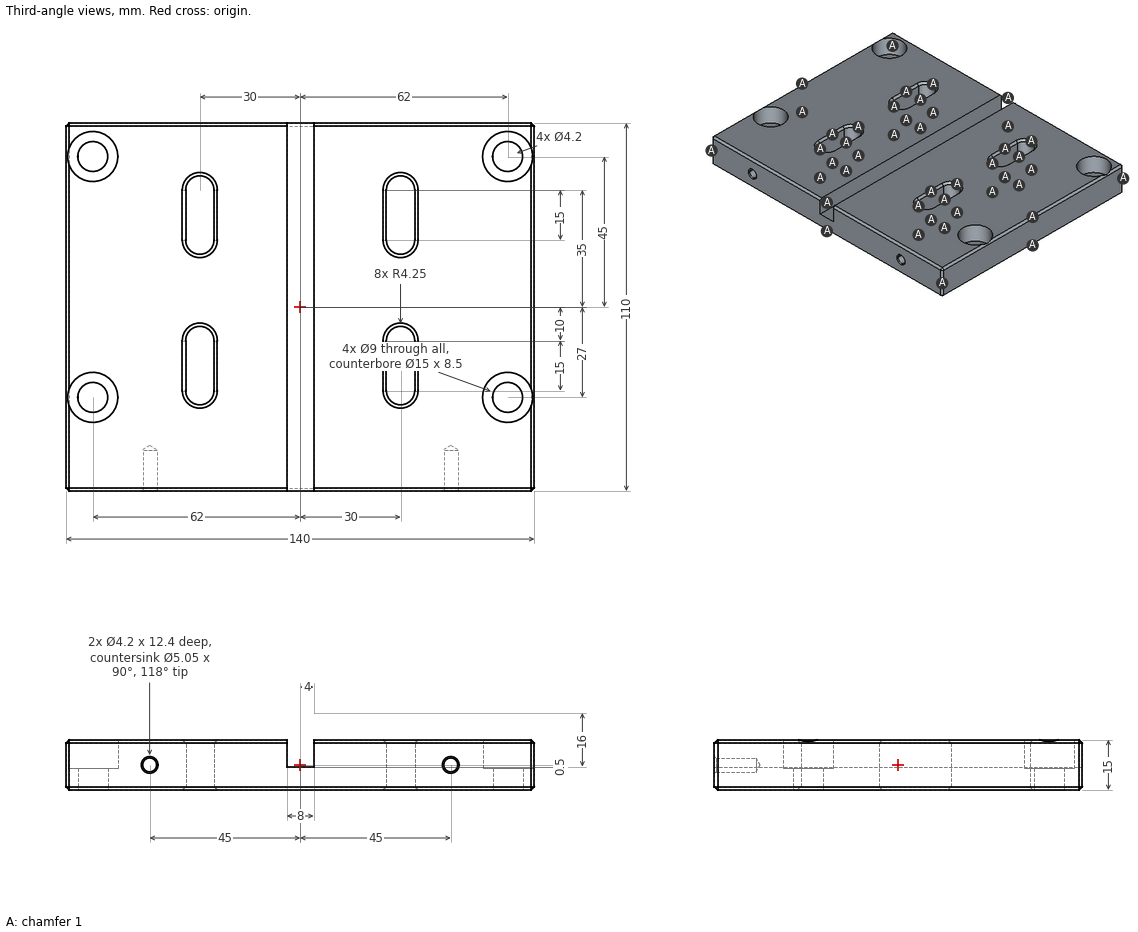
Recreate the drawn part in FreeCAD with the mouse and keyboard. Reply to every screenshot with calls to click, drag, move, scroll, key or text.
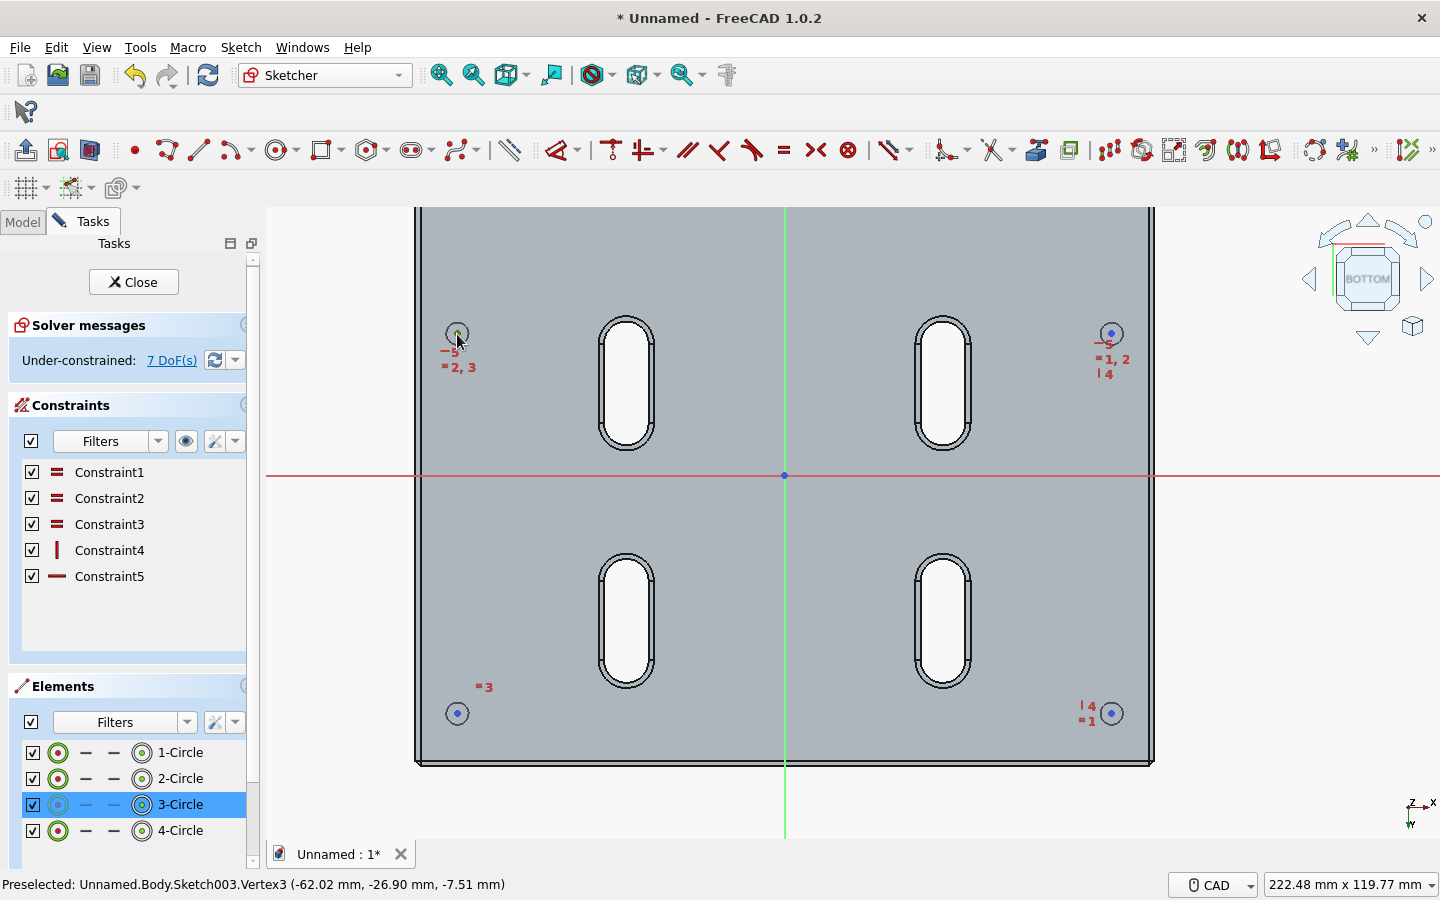
click(457, 714)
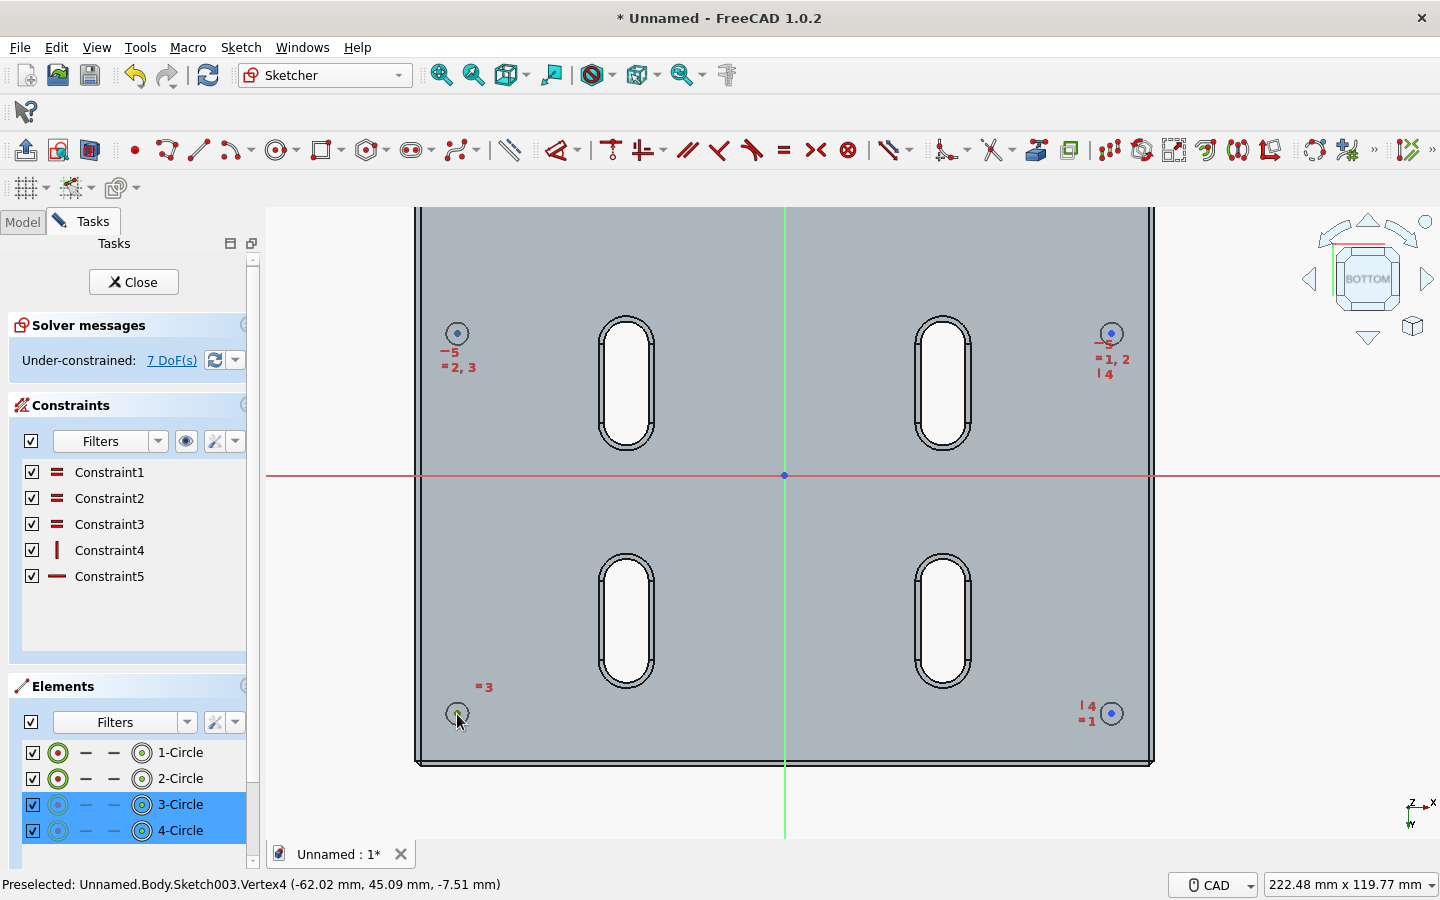
key(v)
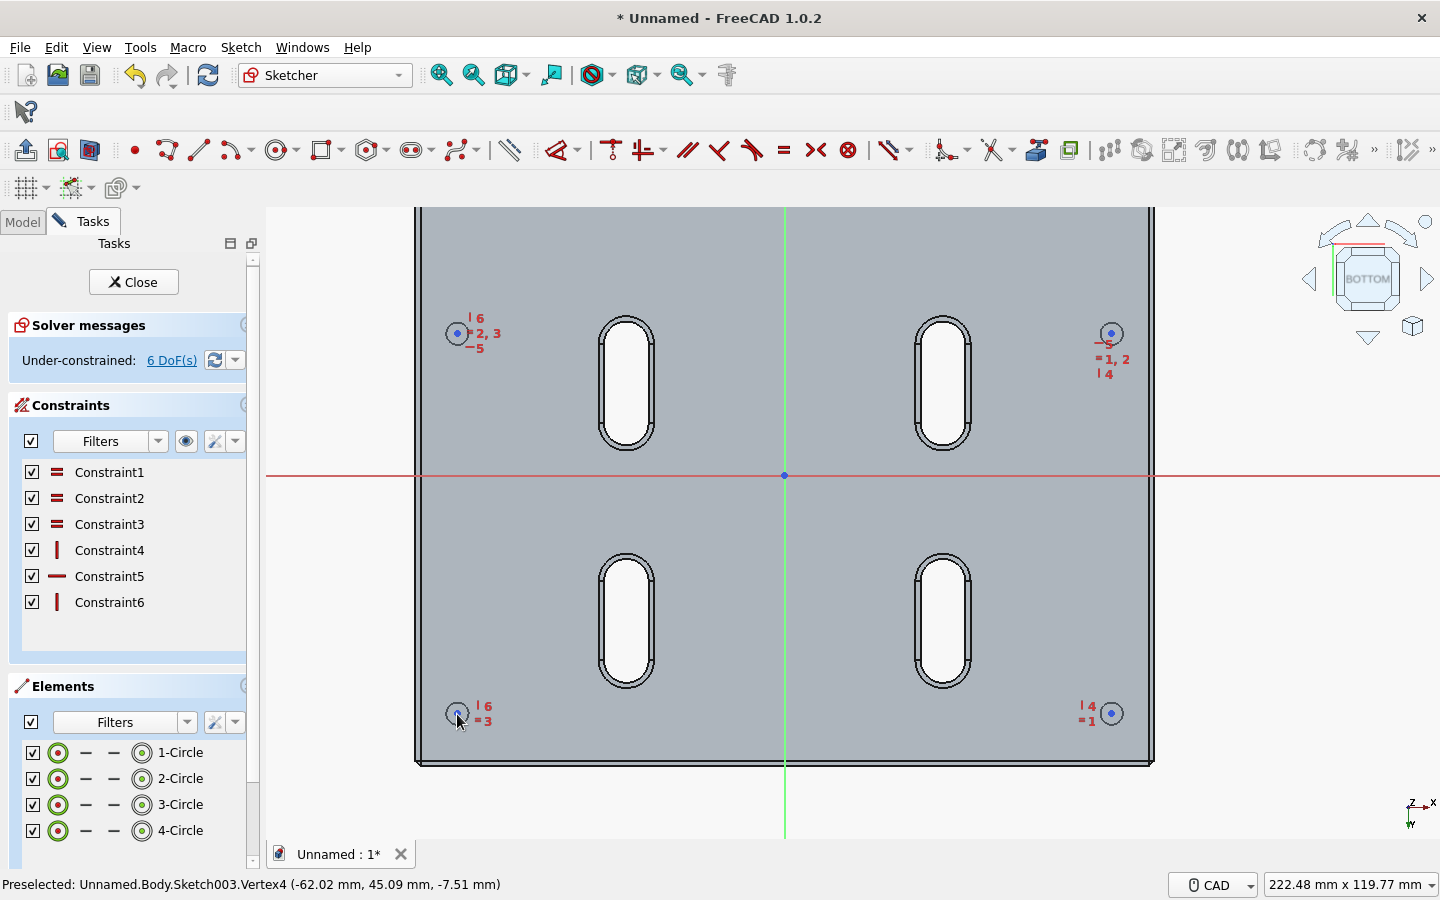
click(1112, 714)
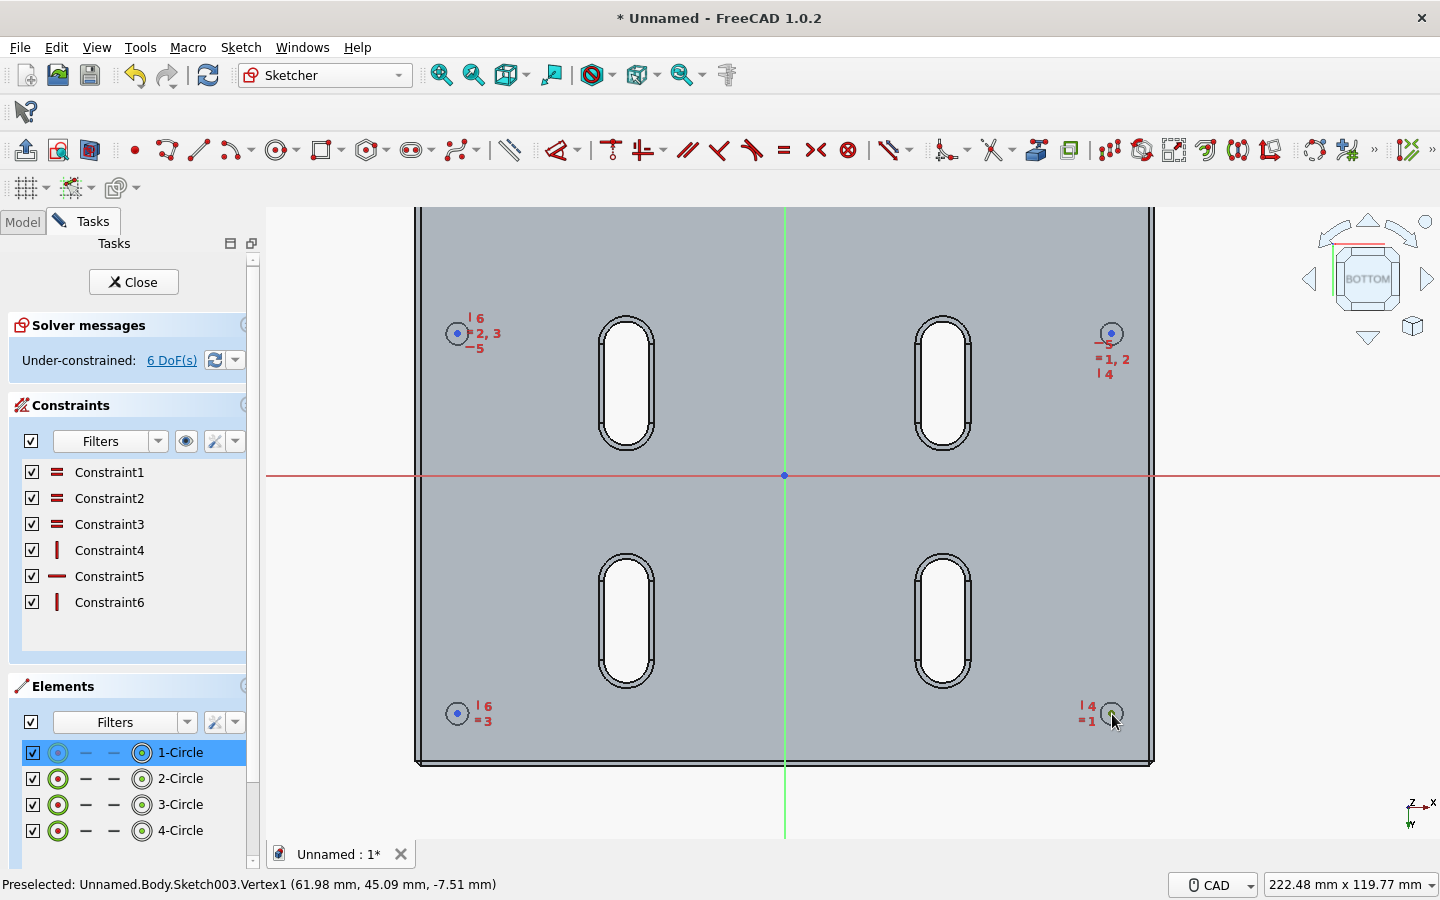
click(457, 714)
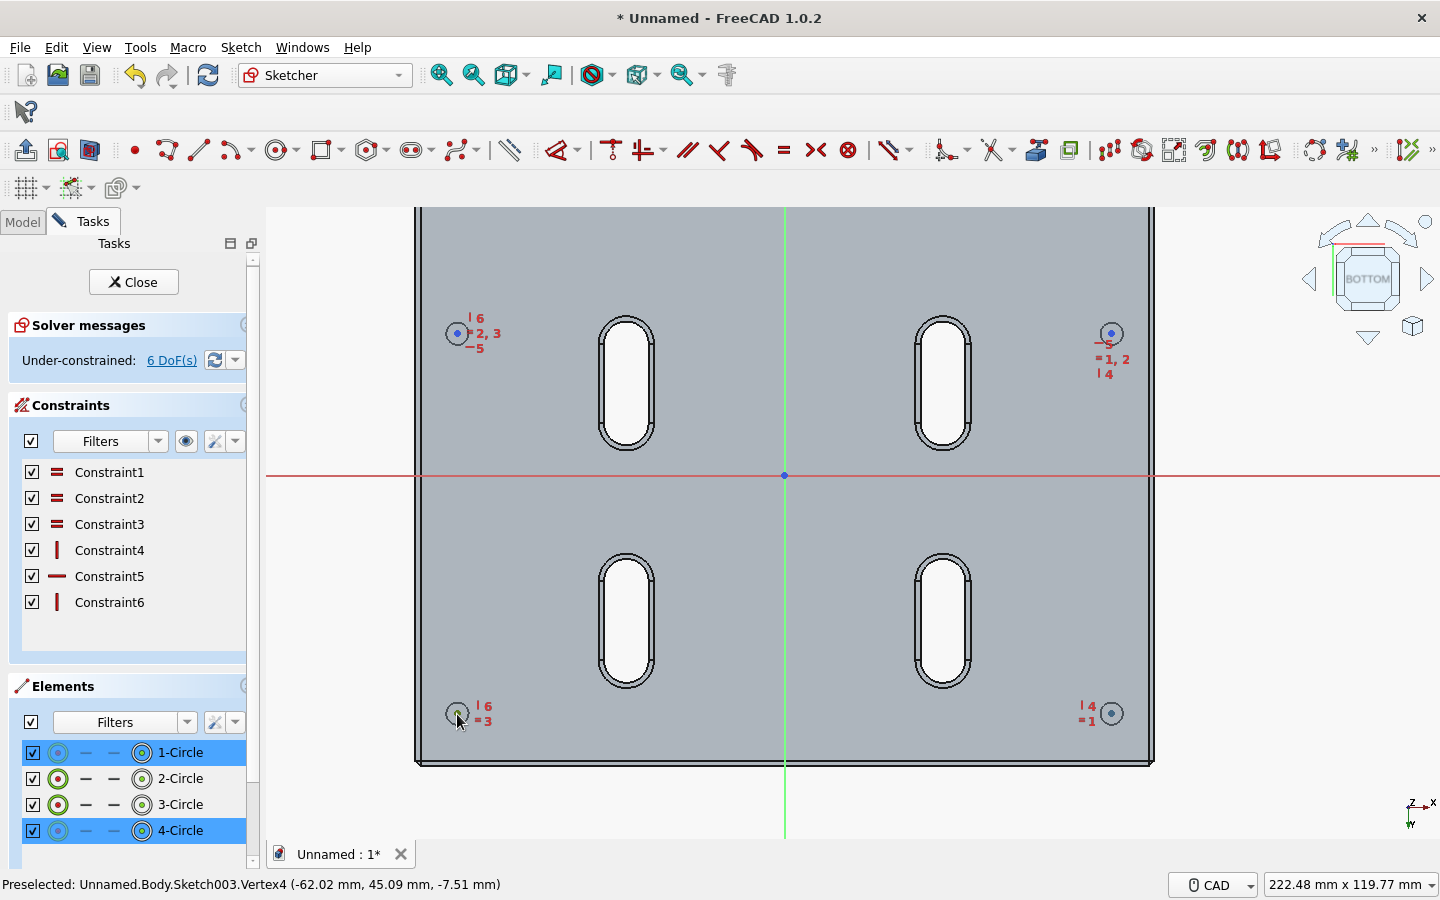
key(h)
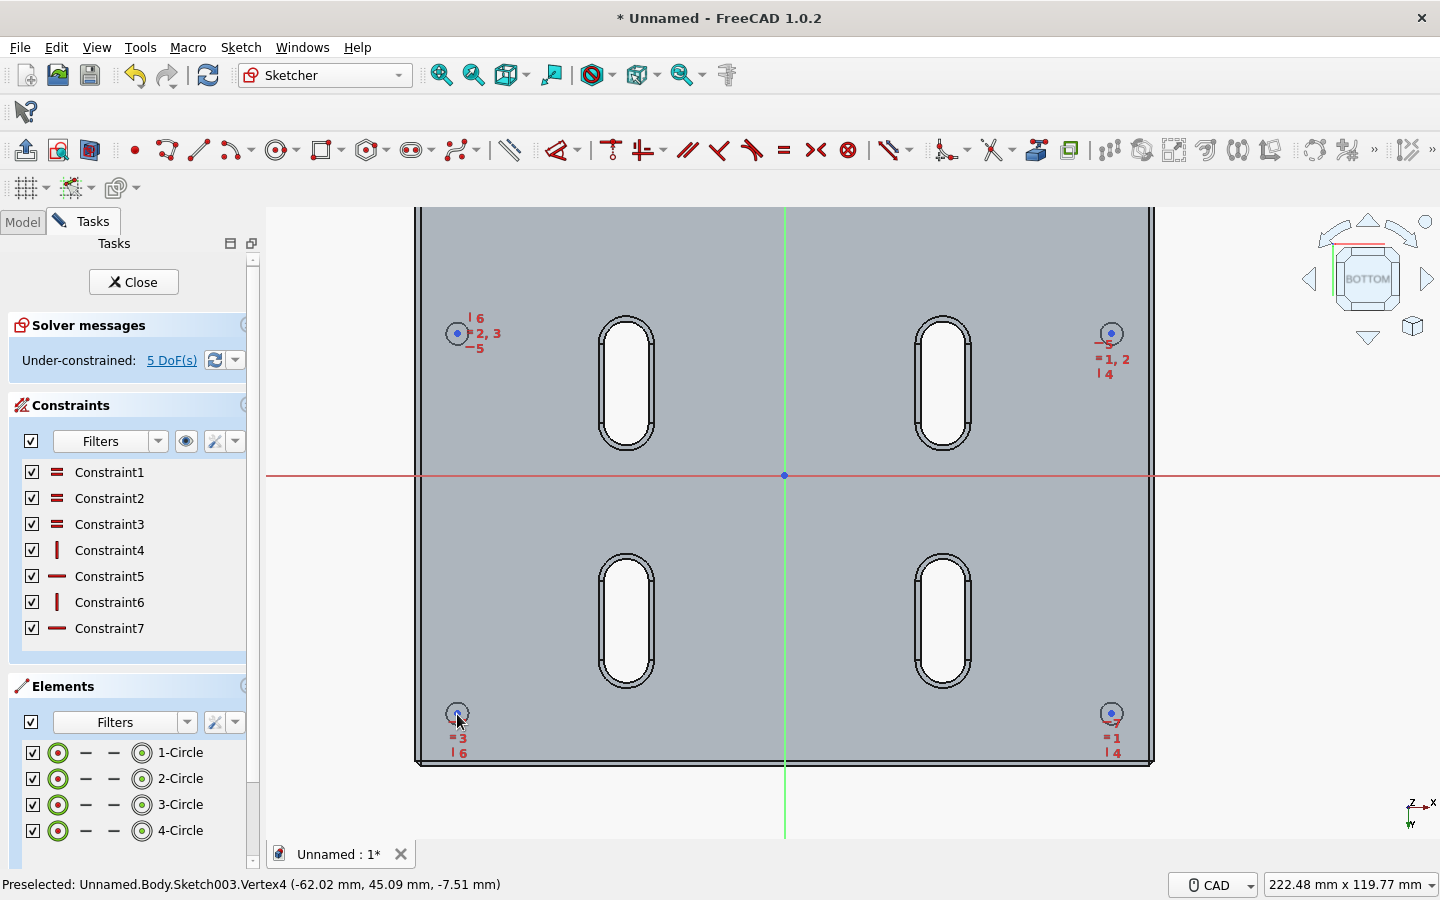
click(556, 150)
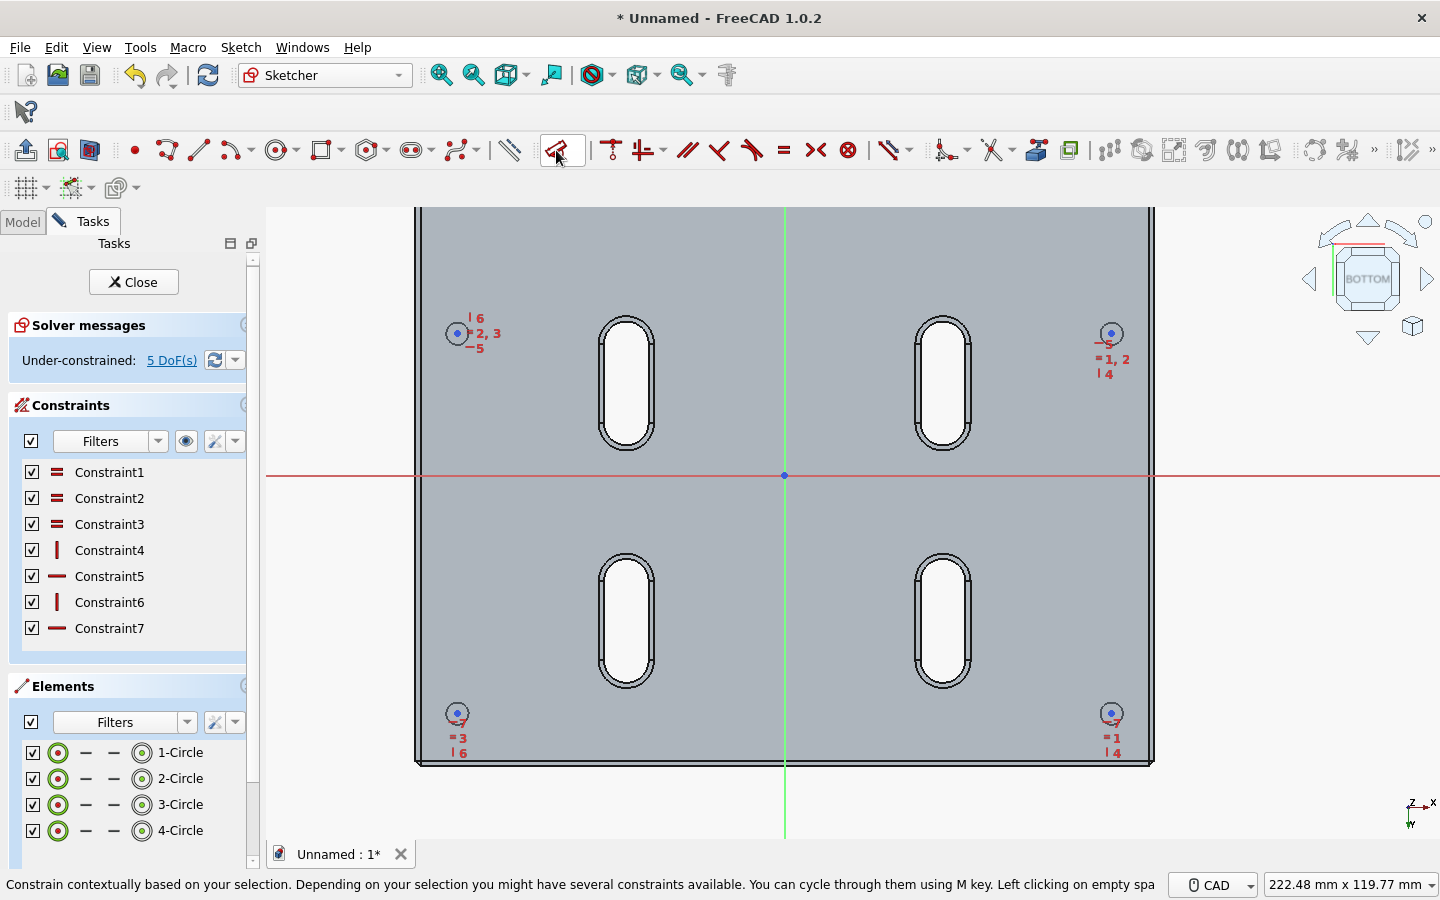
scroll(1120, 706, up, 3)